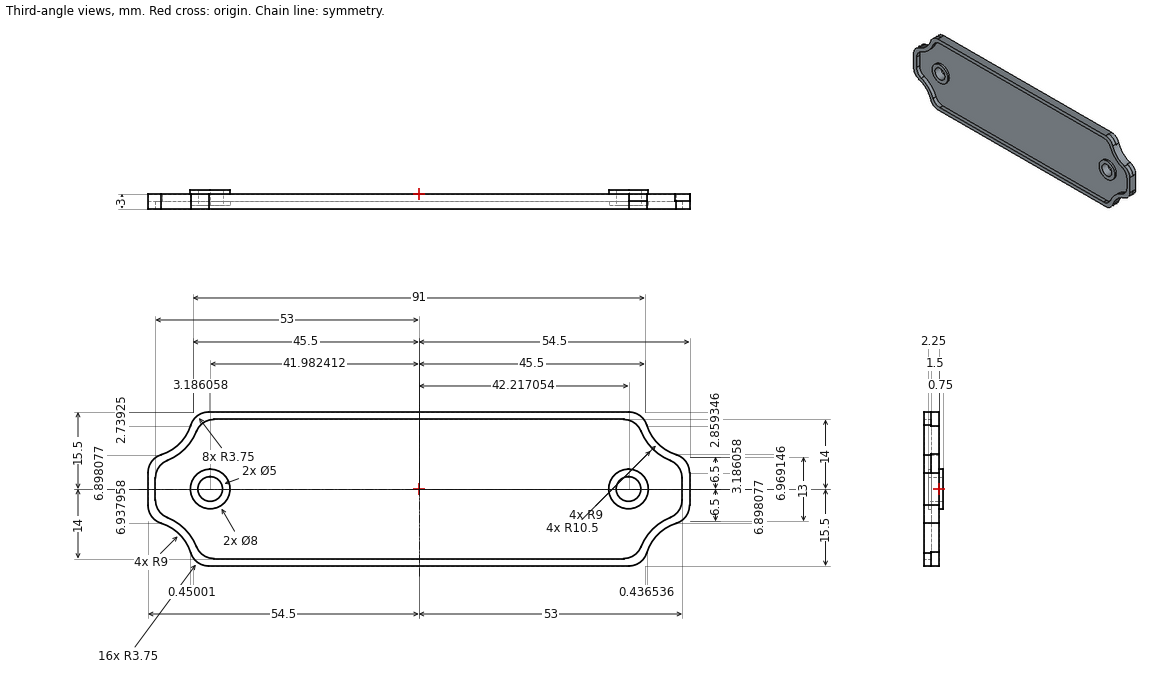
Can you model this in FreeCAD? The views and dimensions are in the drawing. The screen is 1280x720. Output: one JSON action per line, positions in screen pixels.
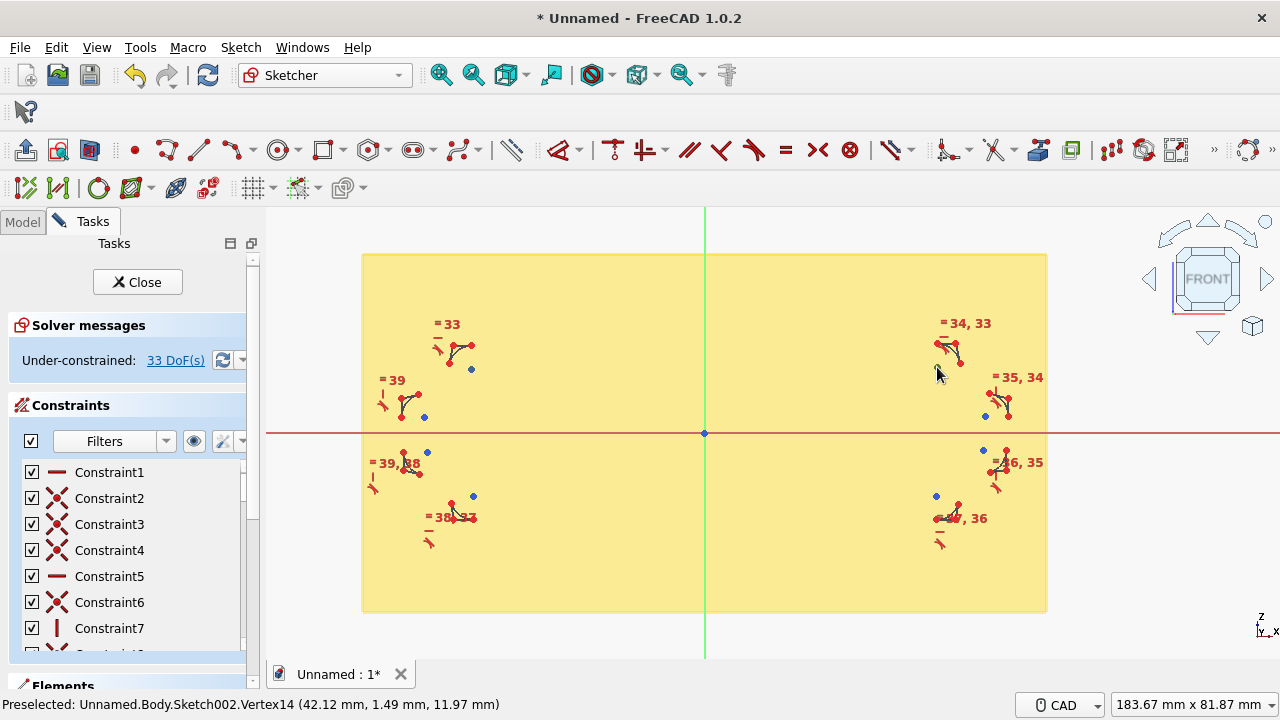
{"action": "left_click", "coordinate": [705, 603]}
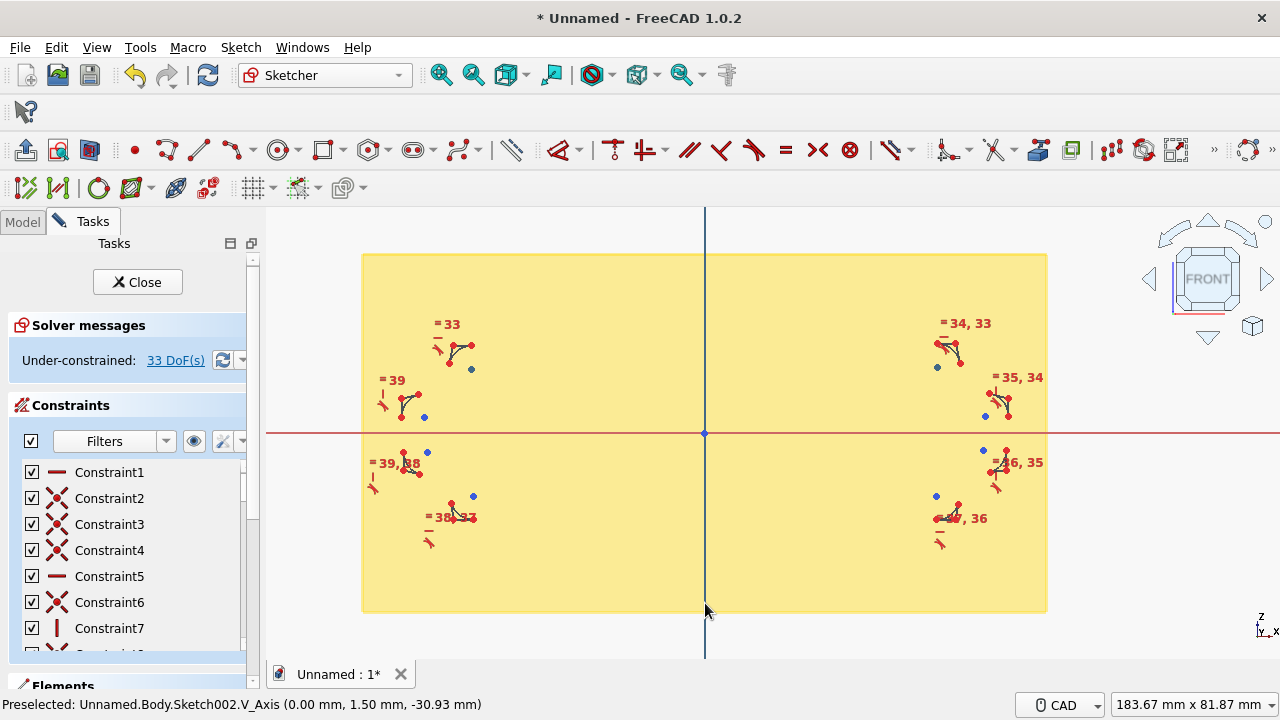
{"action": "left_click", "coordinate": [818, 150]}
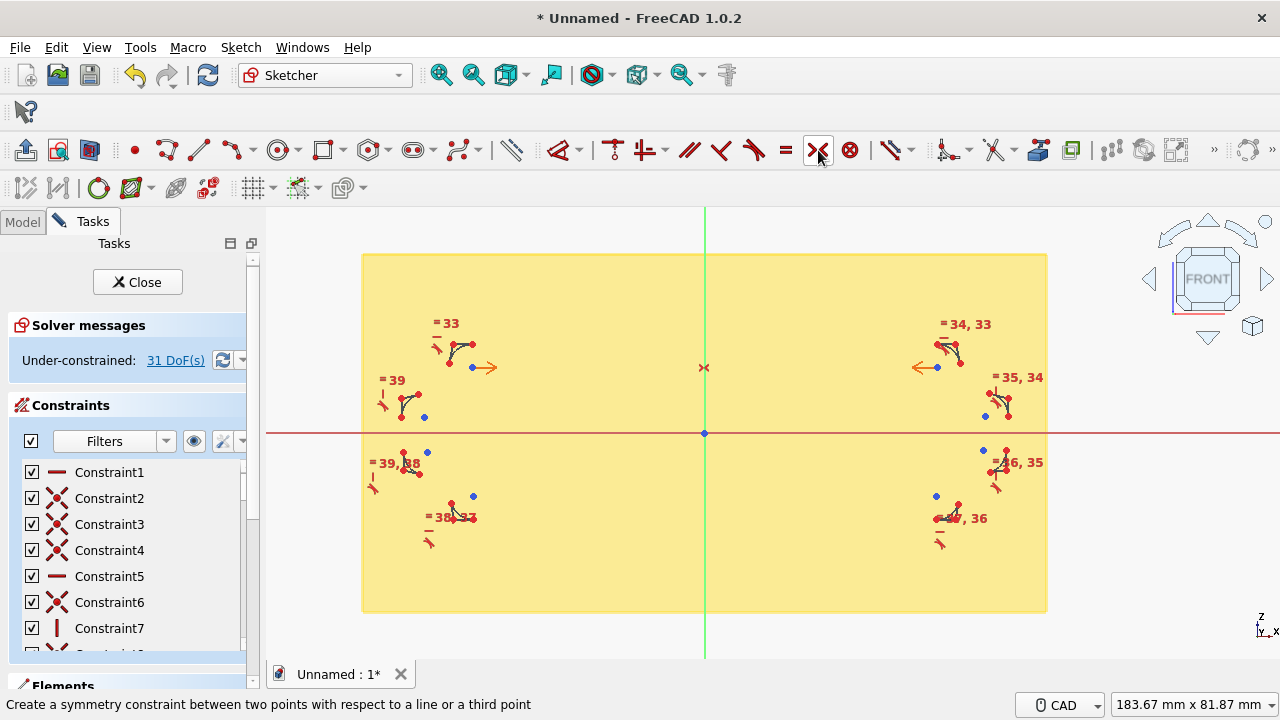
{"action": "left_click", "coordinate": [985, 416]}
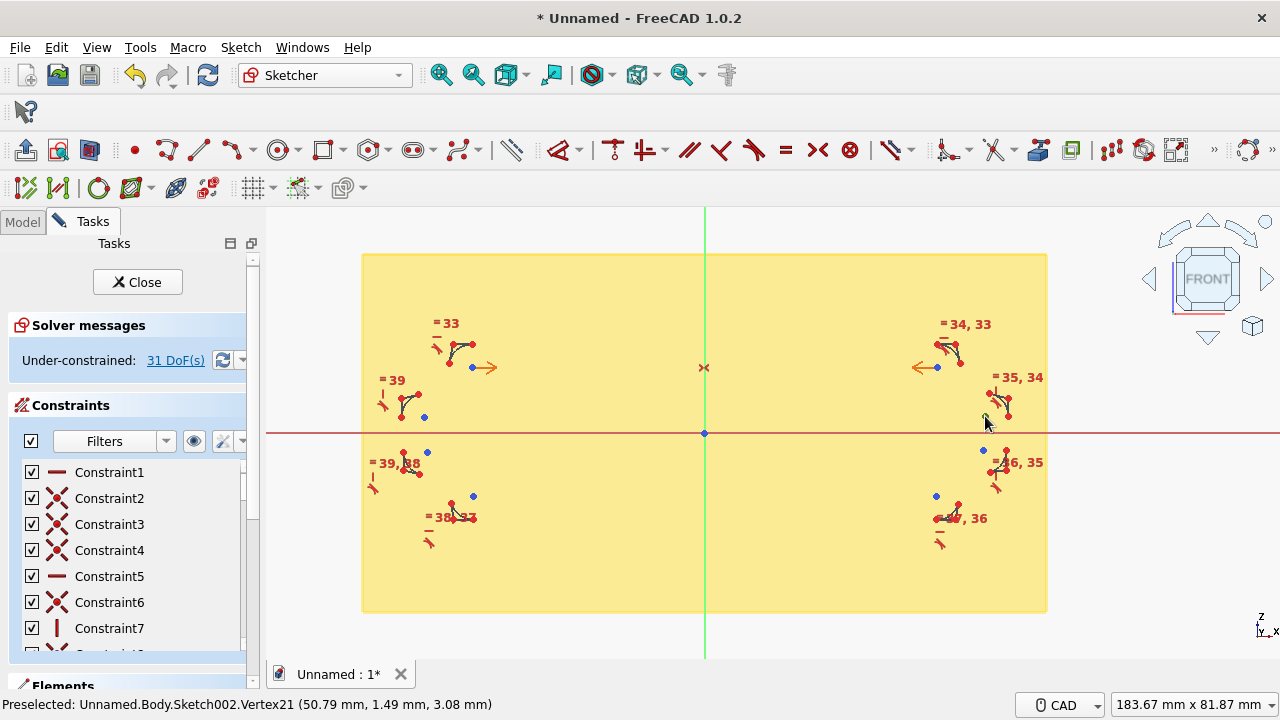
{"action": "left_click", "coordinate": [983, 450]}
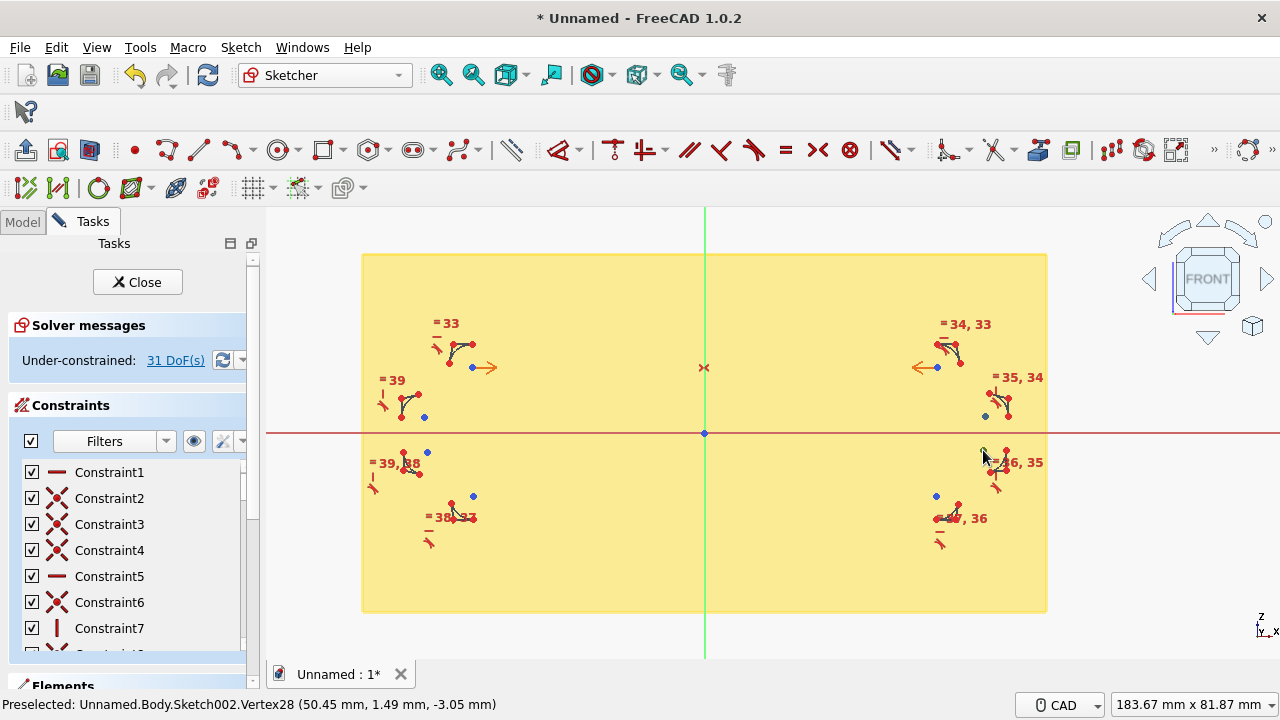
{"action": "left_click", "coordinate": [353, 433]}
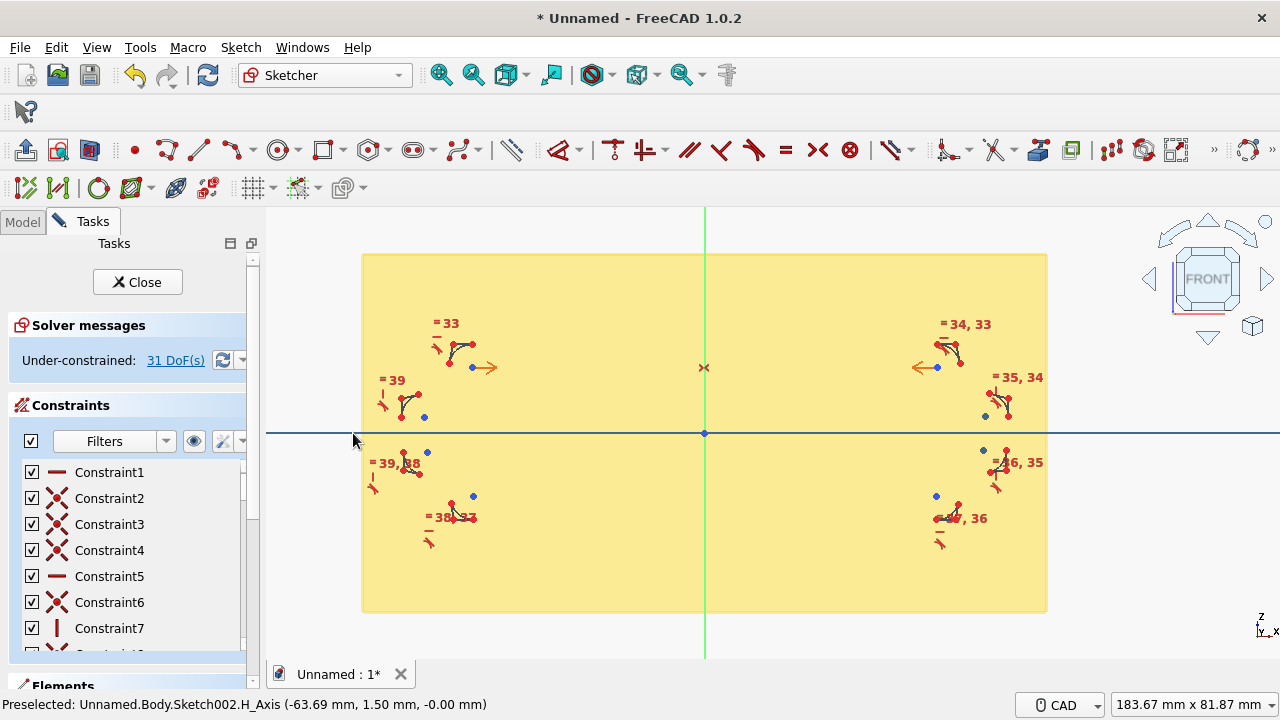
{"action": "left_click", "coordinate": [818, 150]}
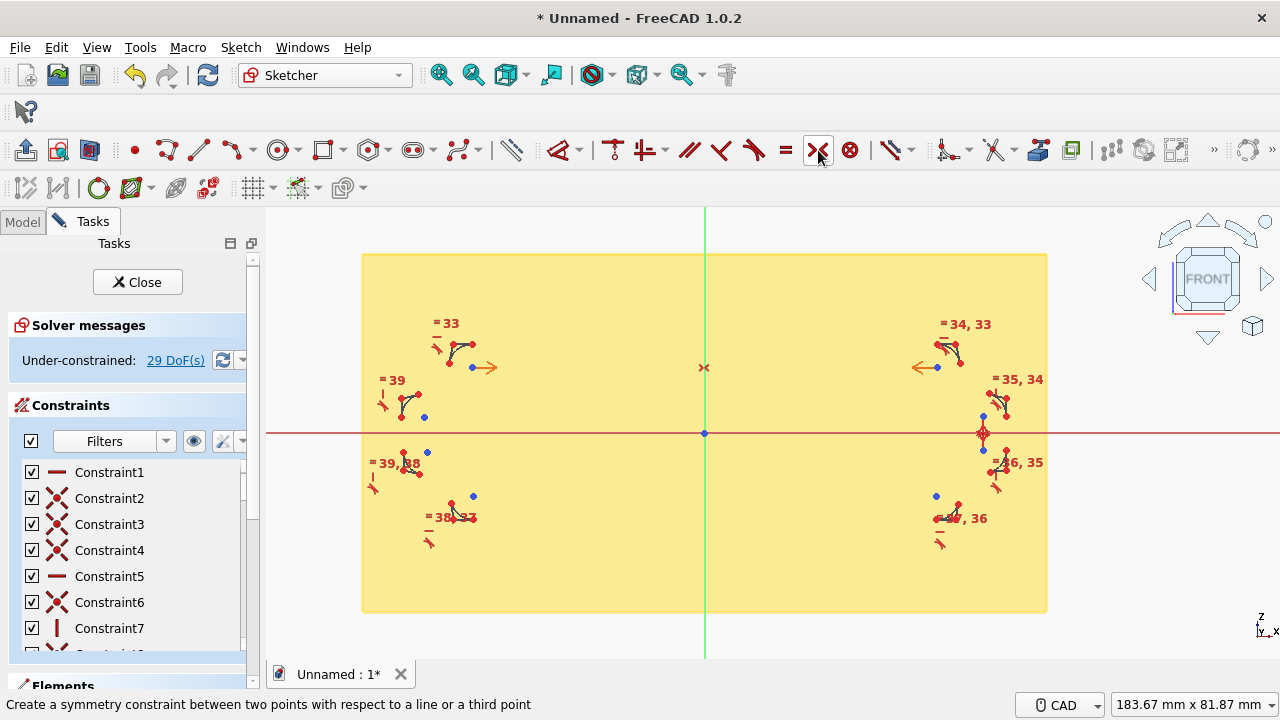
{"action": "left_click", "coordinate": [937, 368]}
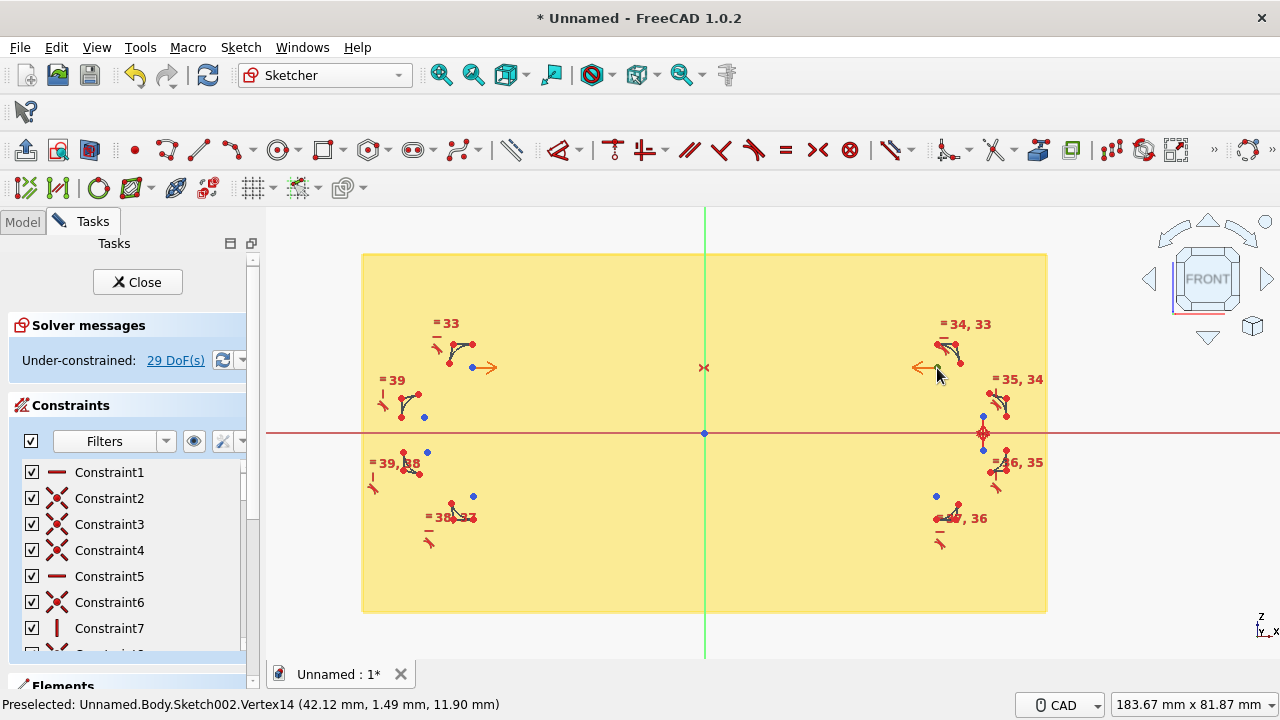
{"action": "left_click", "coordinate": [936, 497]}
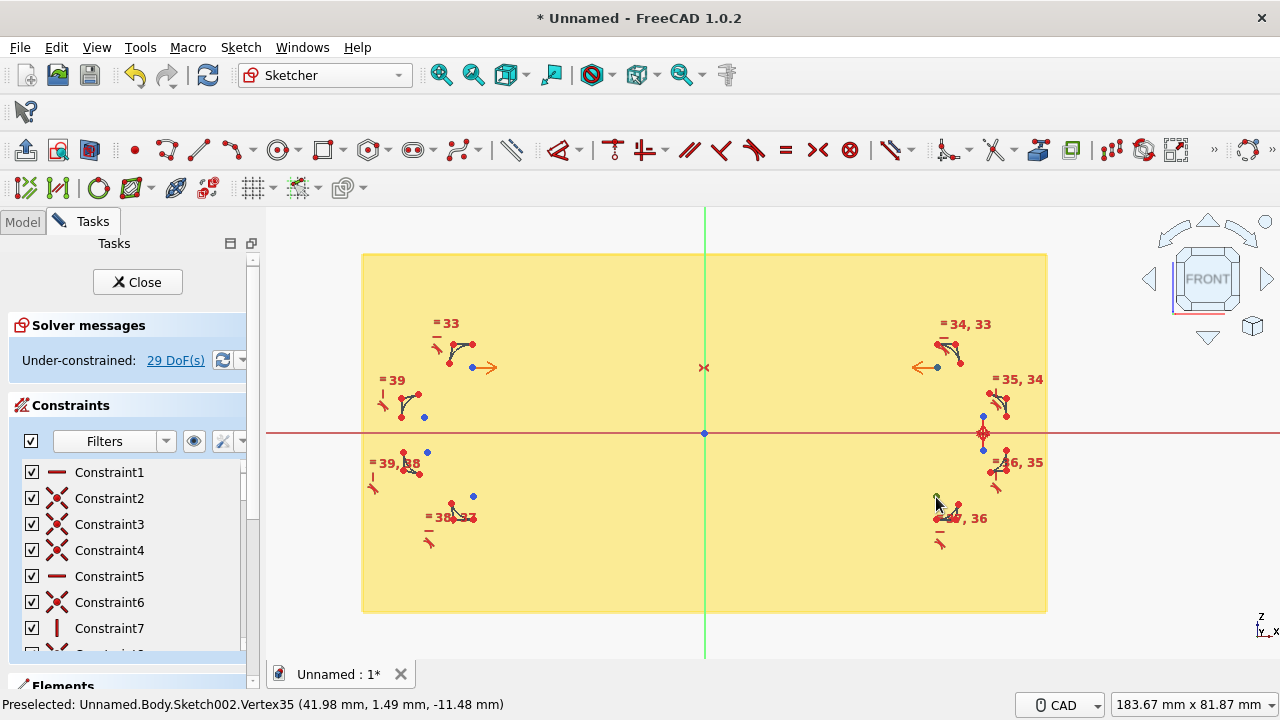
{"action": "left_click", "coordinate": [353, 433]}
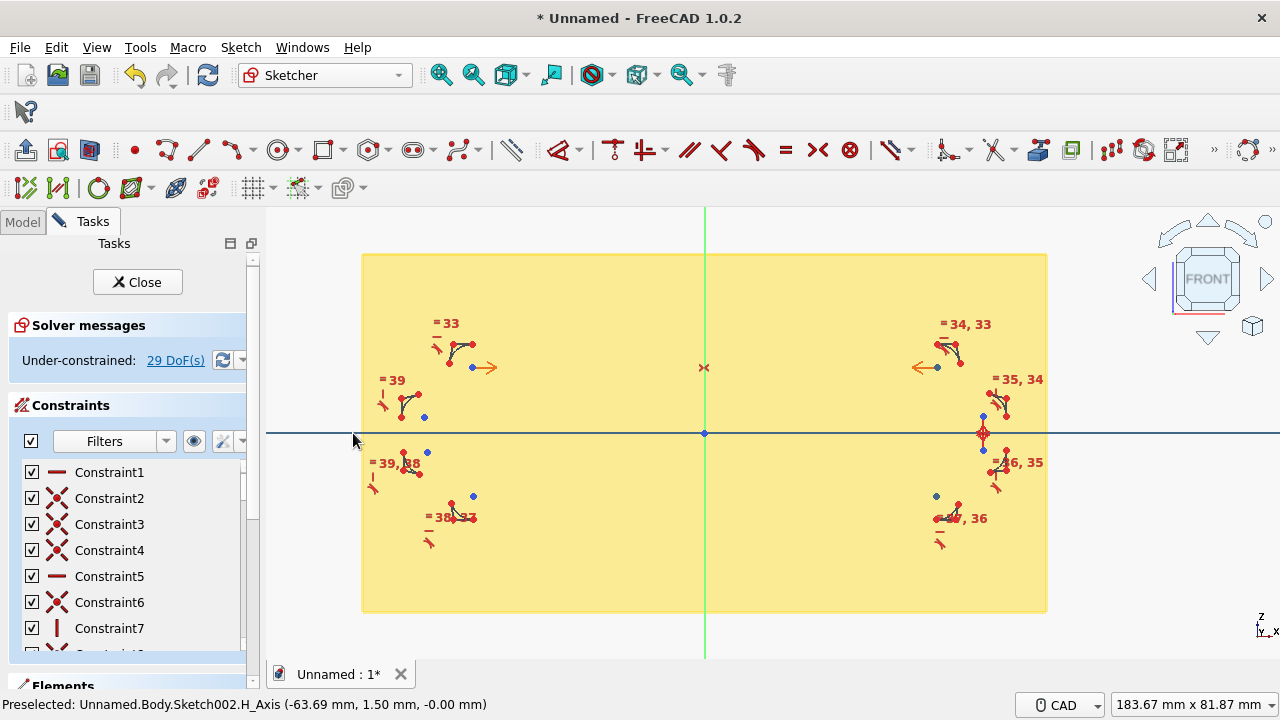
{"action": "left_click", "coordinate": [818, 150]}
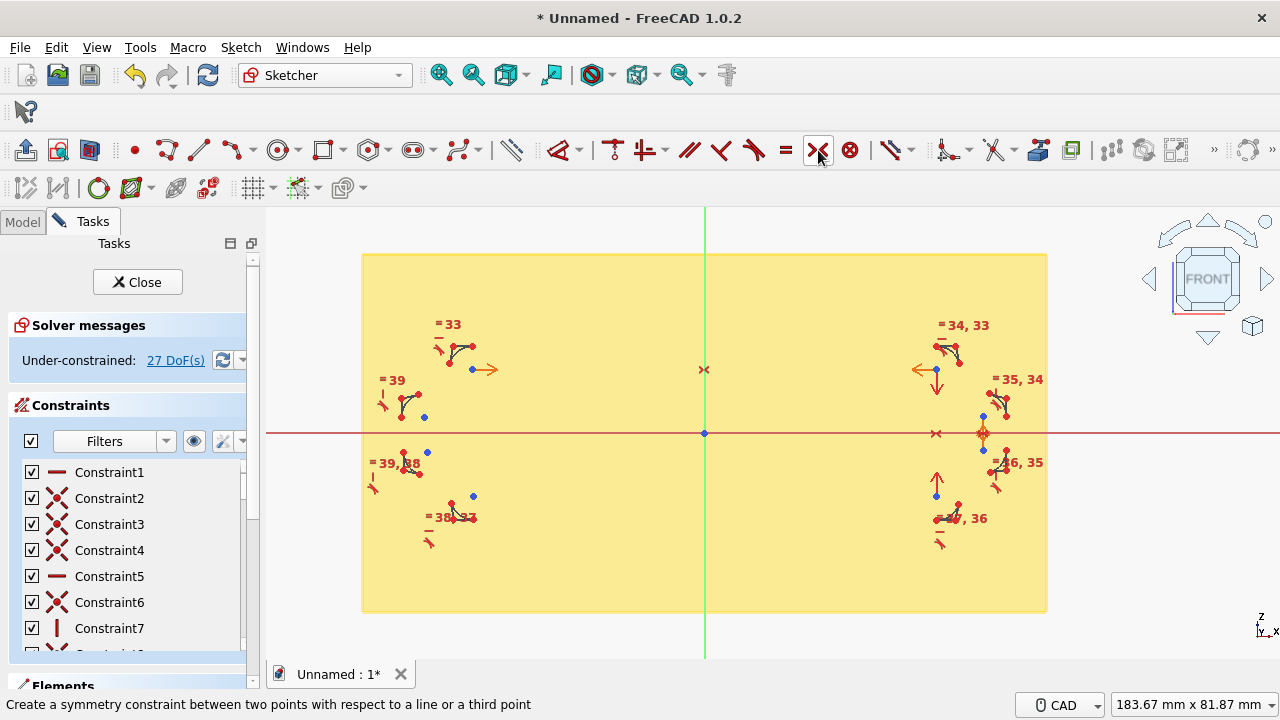
{"action": "left_click", "coordinate": [472, 370]}